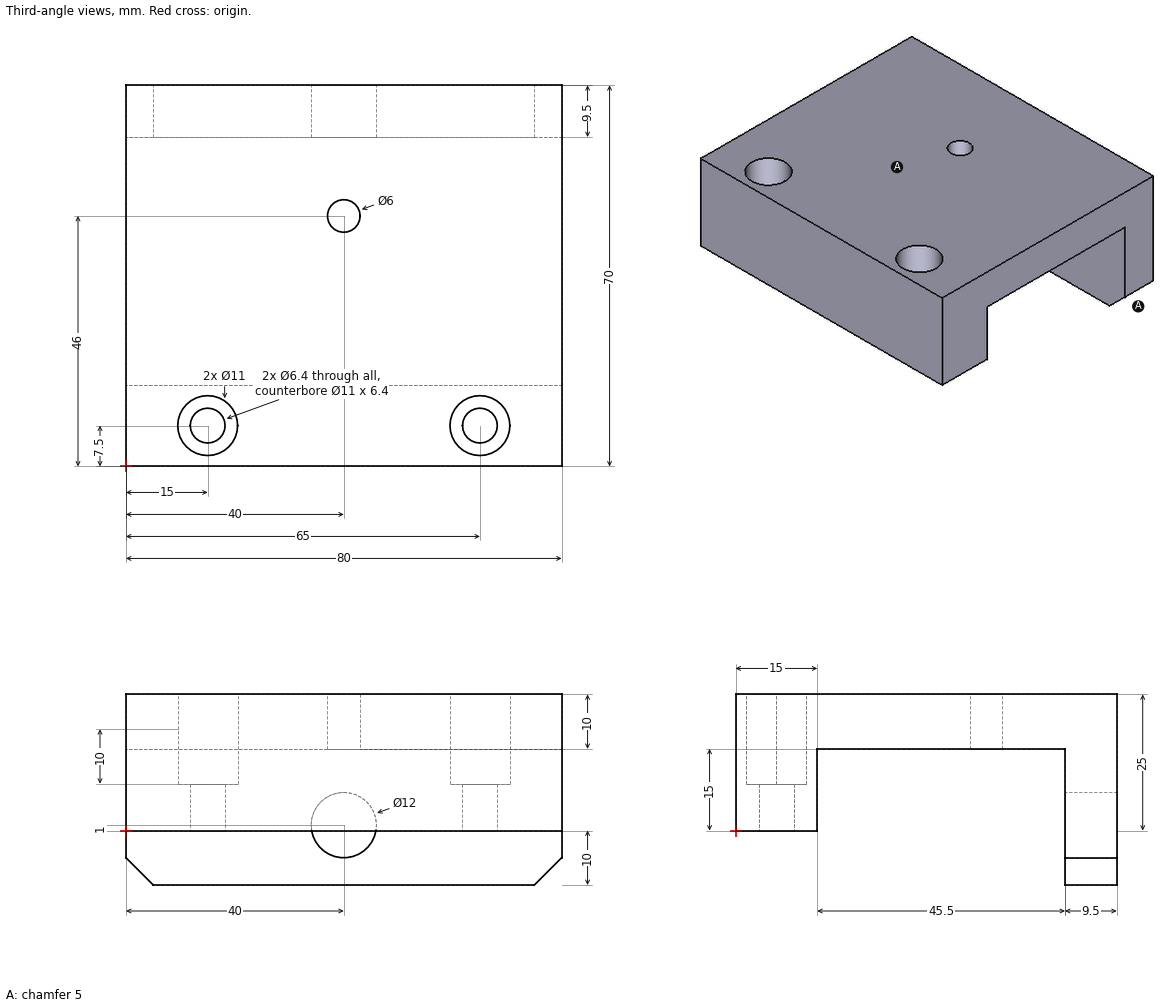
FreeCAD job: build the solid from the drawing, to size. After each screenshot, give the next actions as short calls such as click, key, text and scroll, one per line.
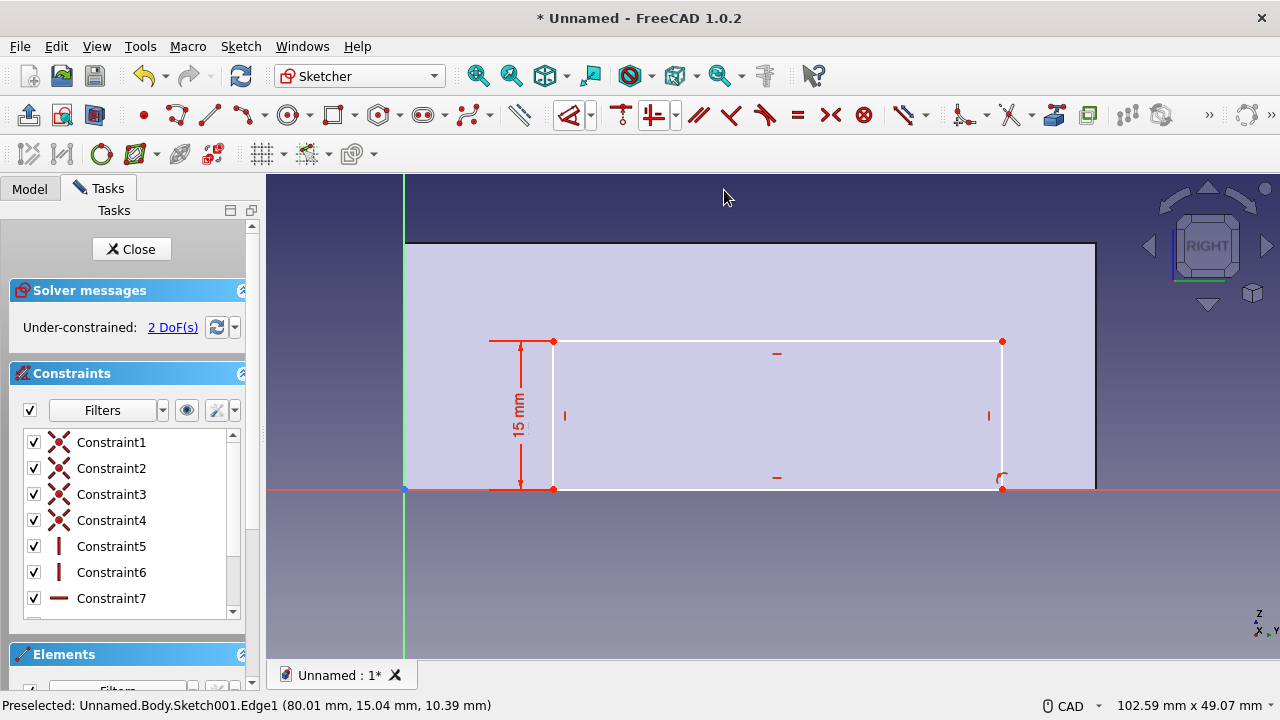
click(553, 341)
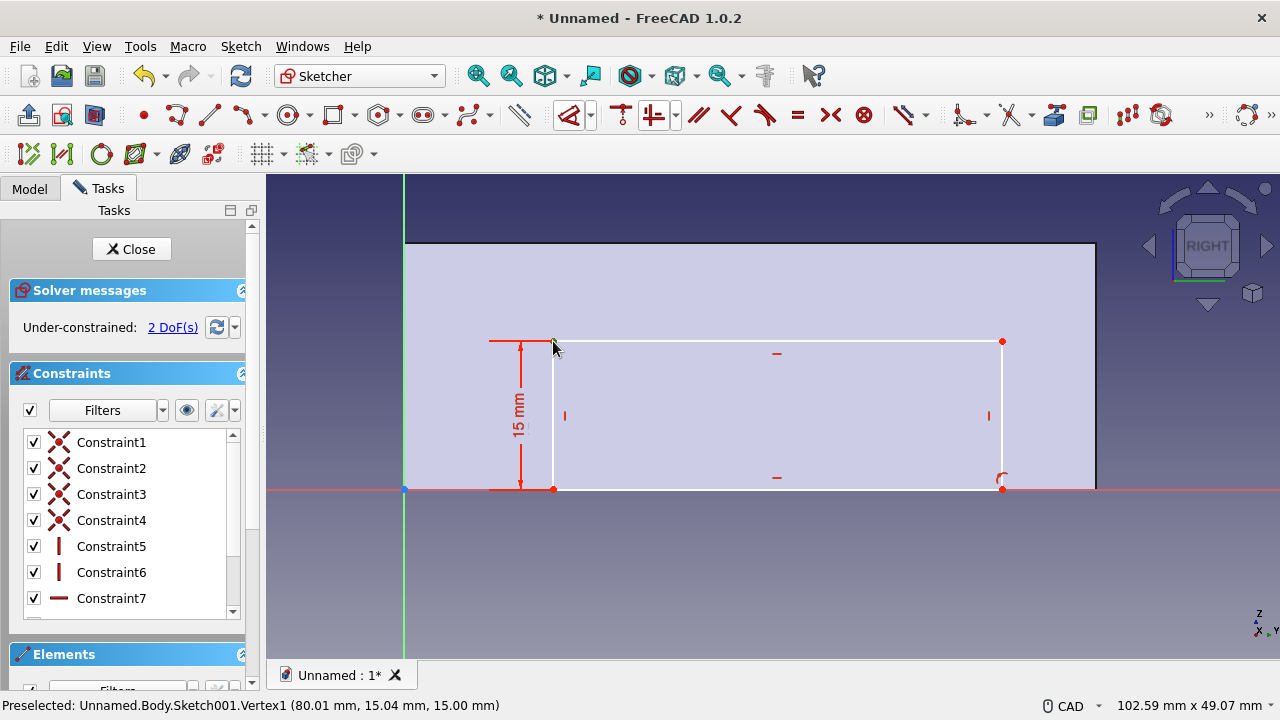
click(590, 116)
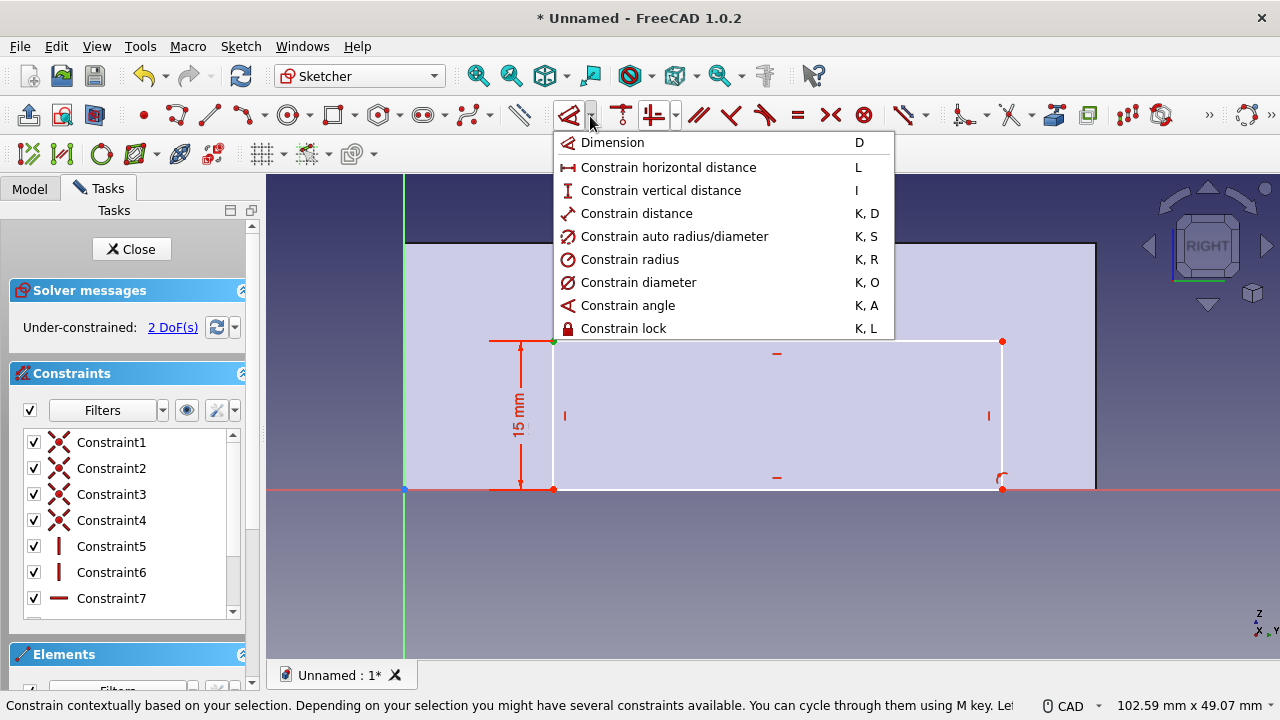
click(724, 168)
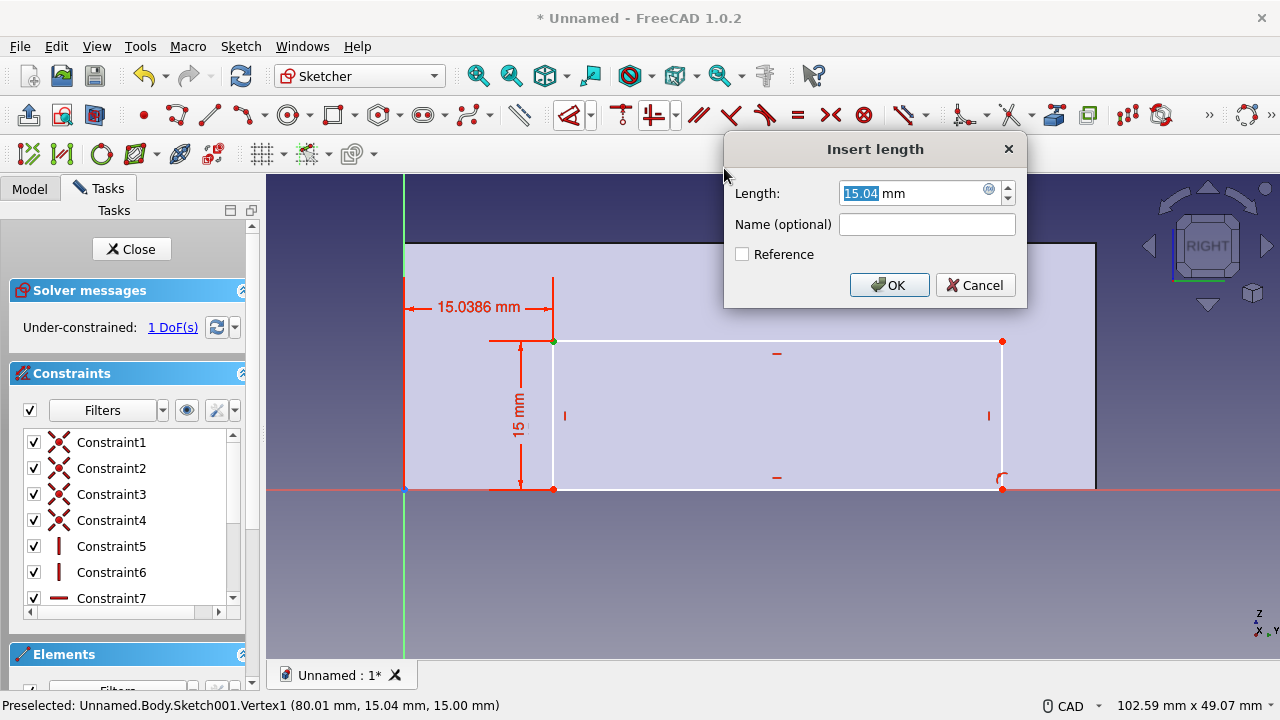
text(15)
key(Return)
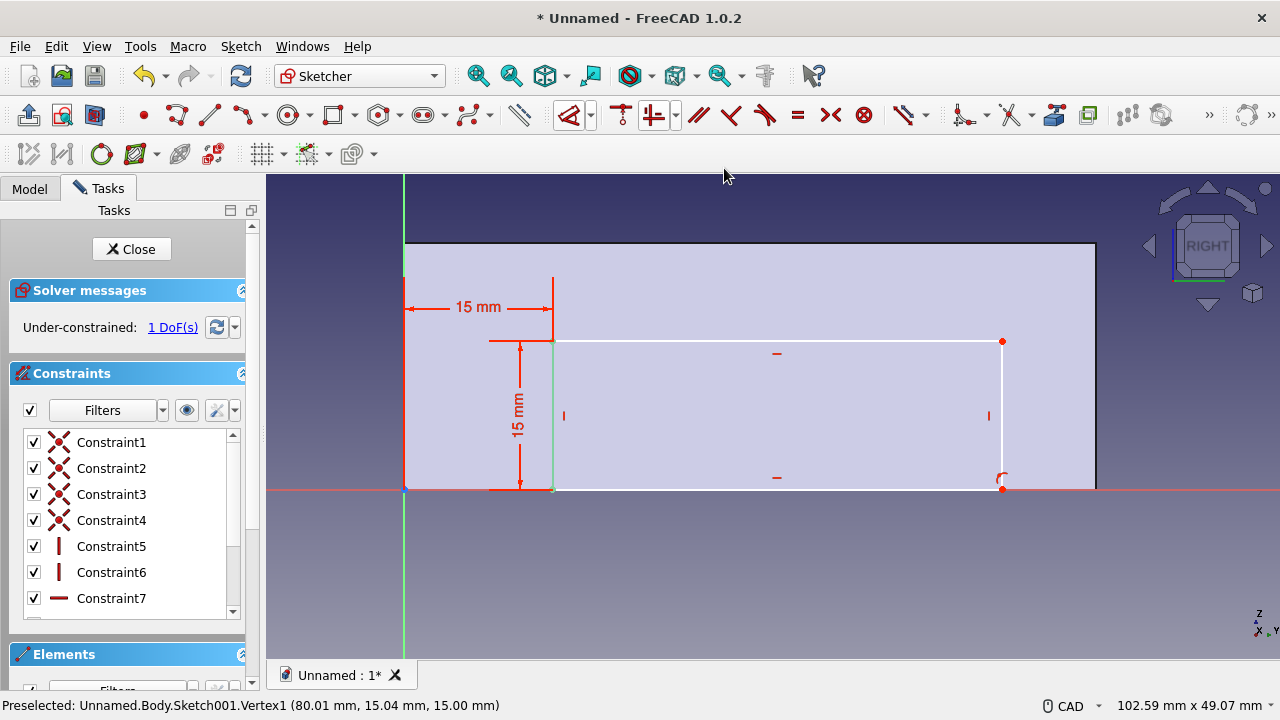
click(687, 490)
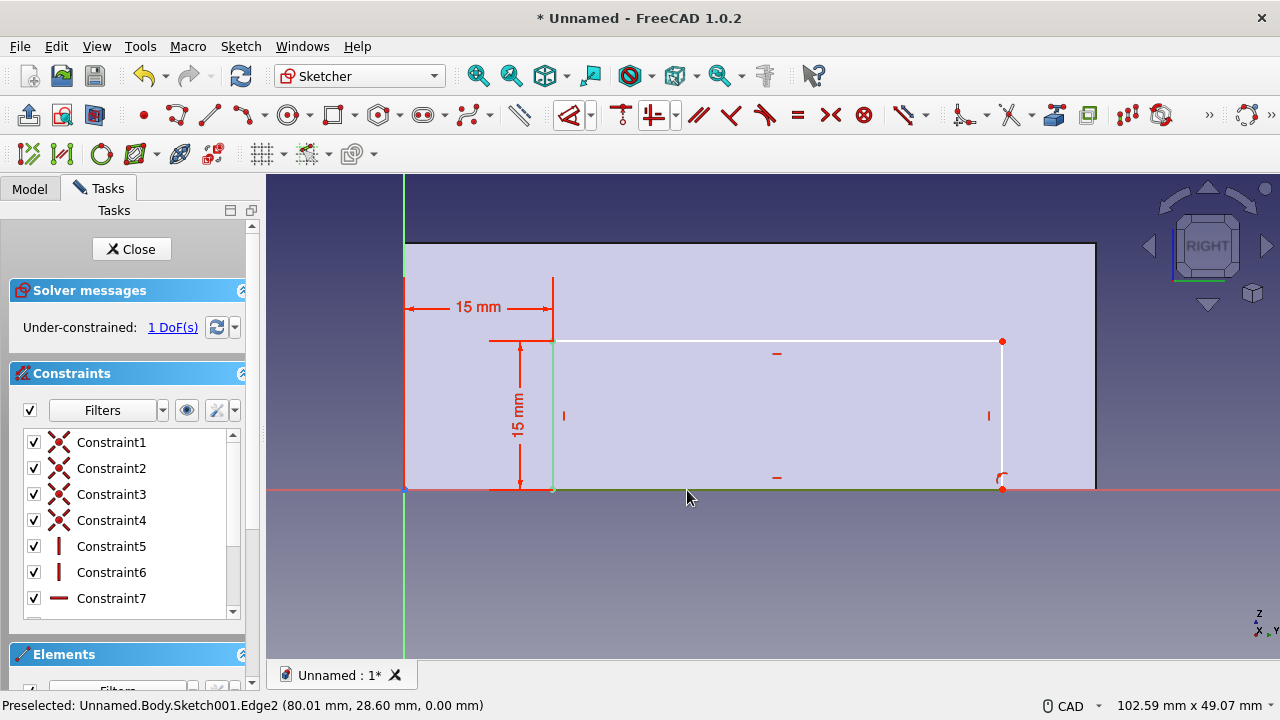
key(l)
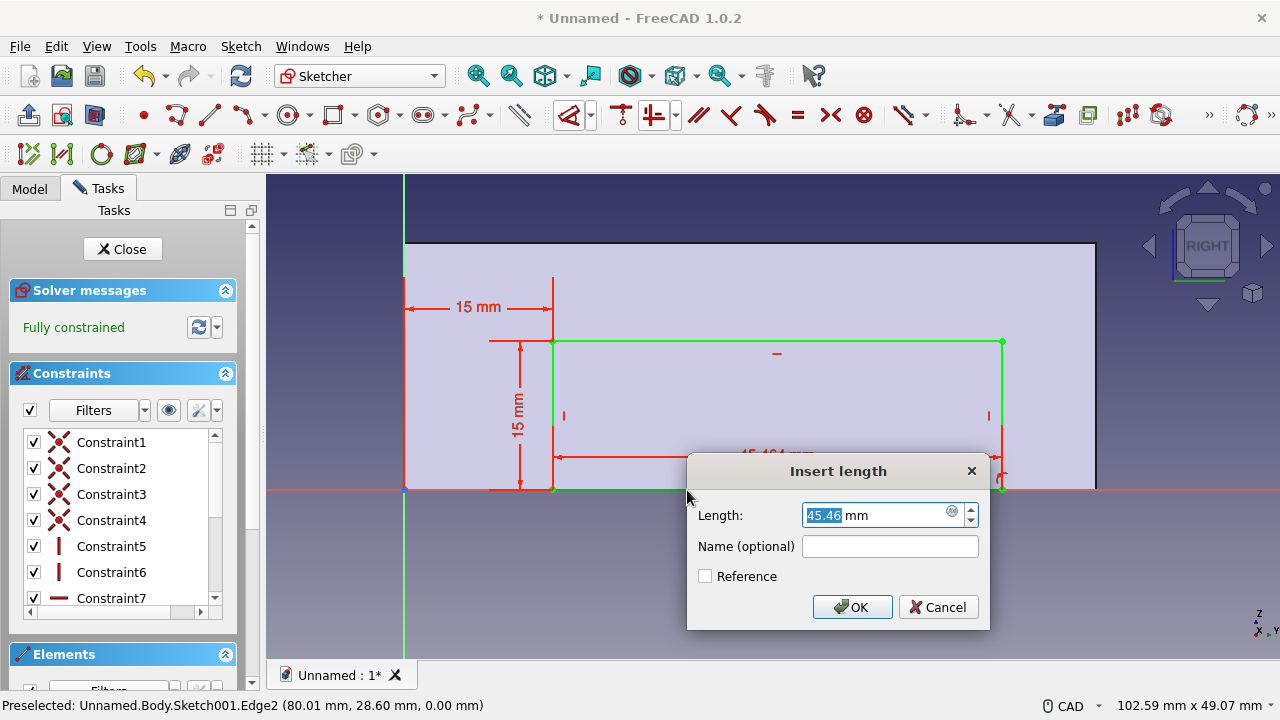
text(45.5)
key(Return)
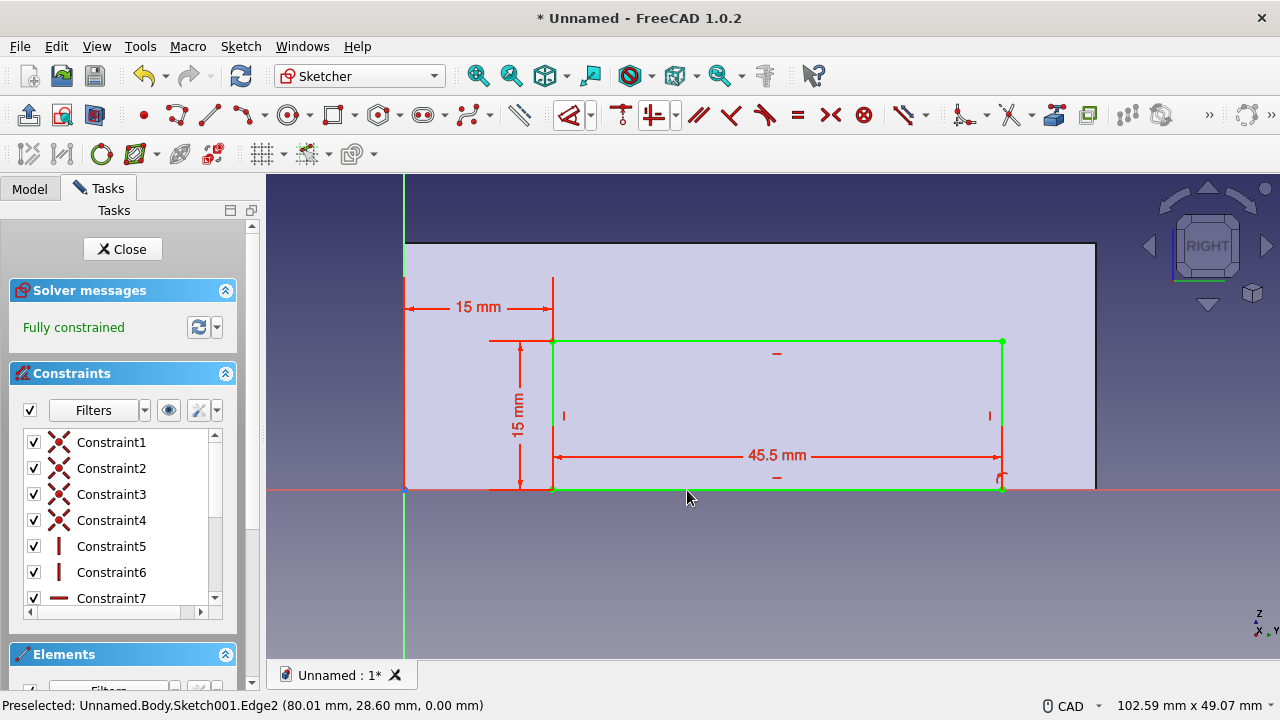
click(123, 249)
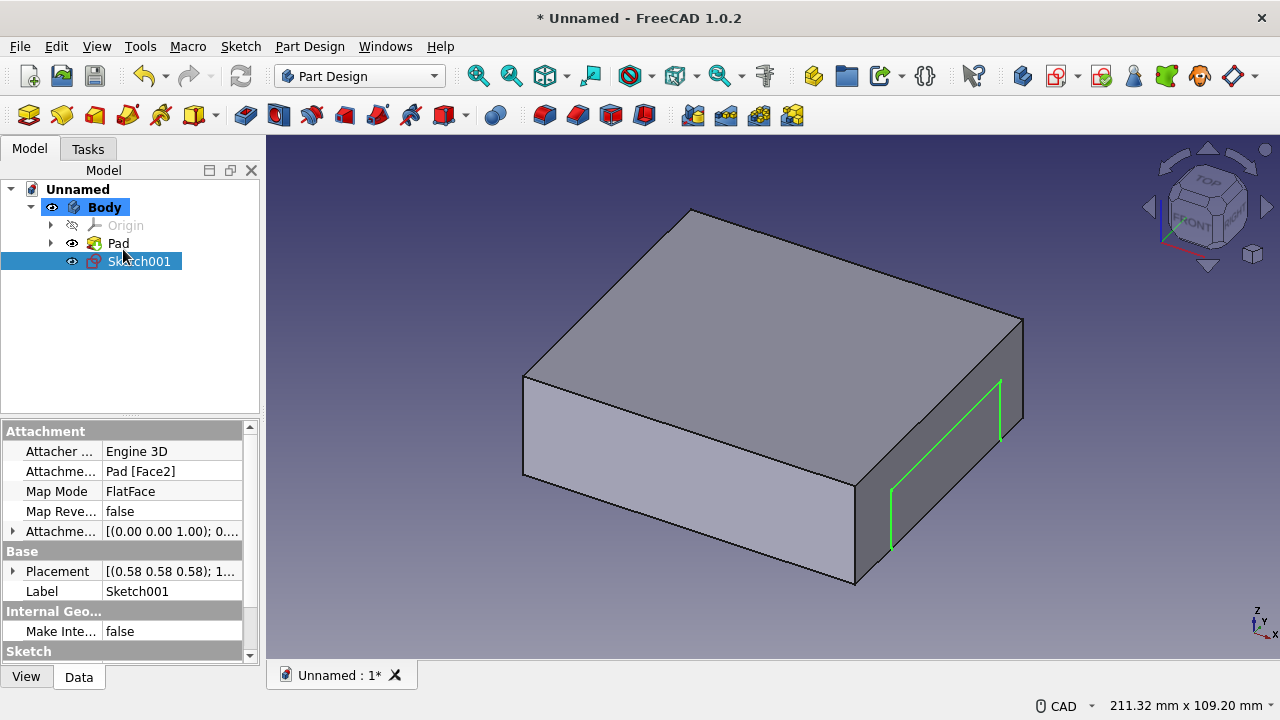
click(246, 116)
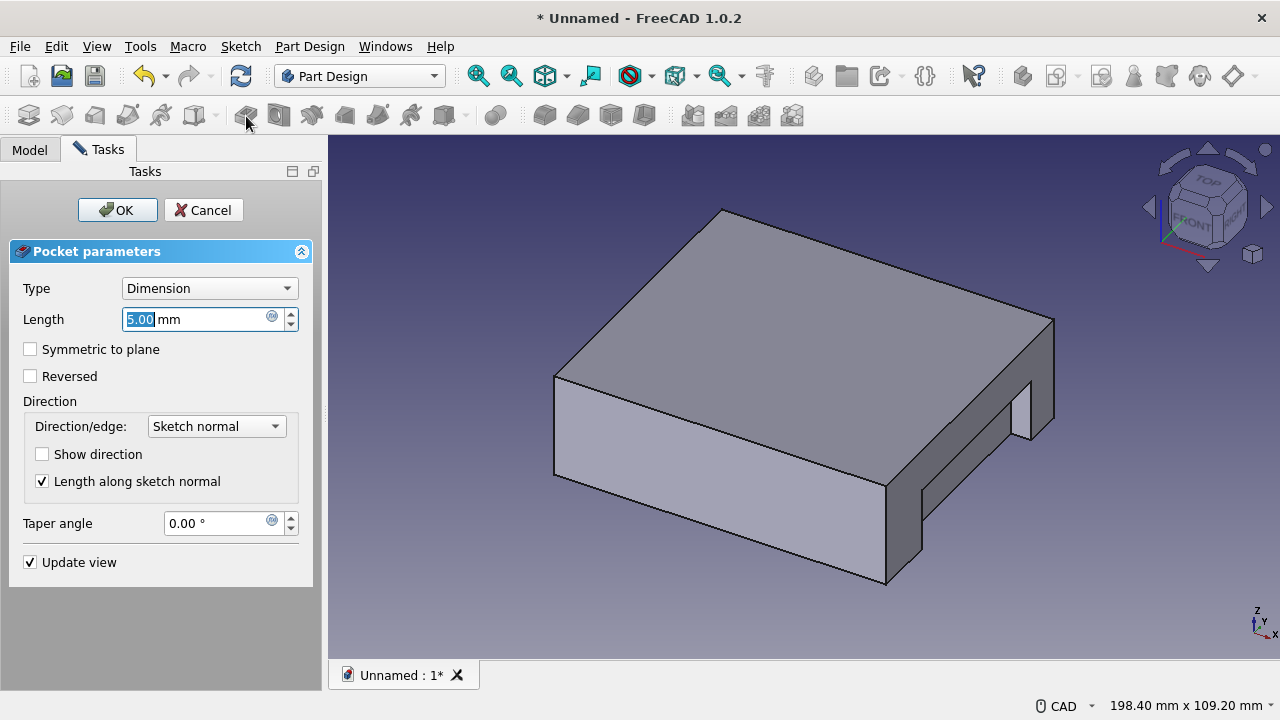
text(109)
key(Tab)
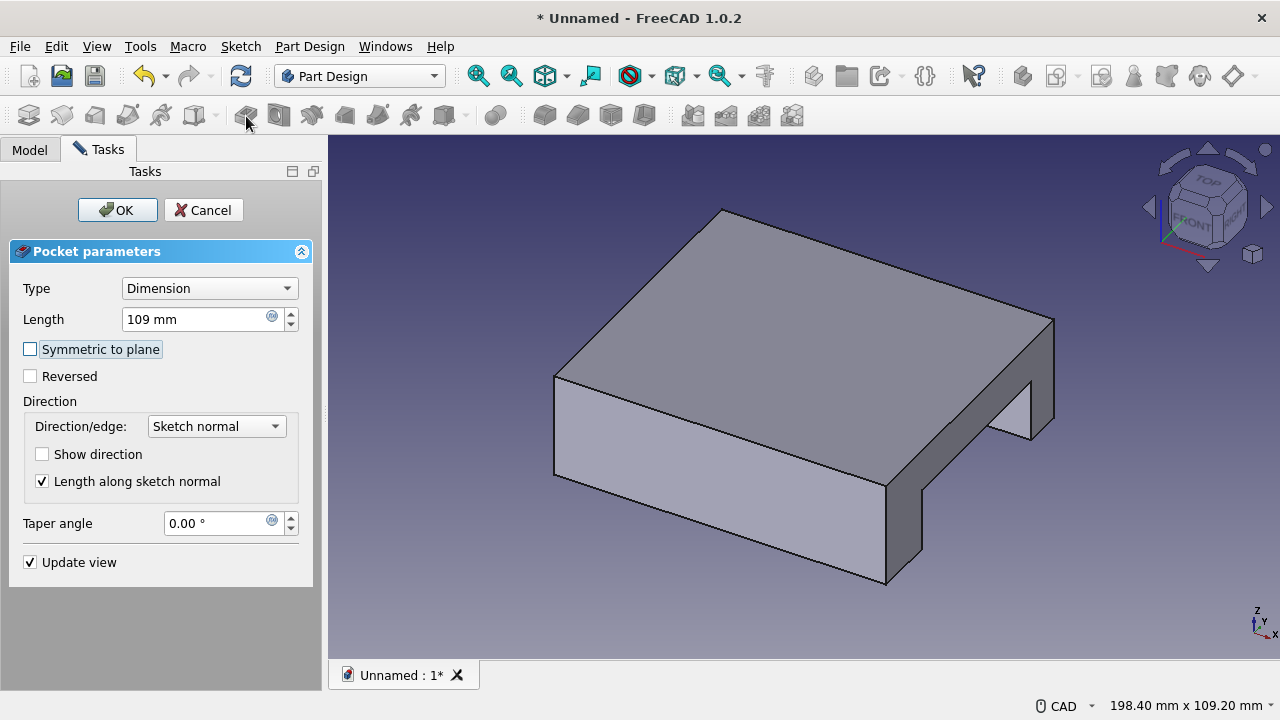
click(118, 210)